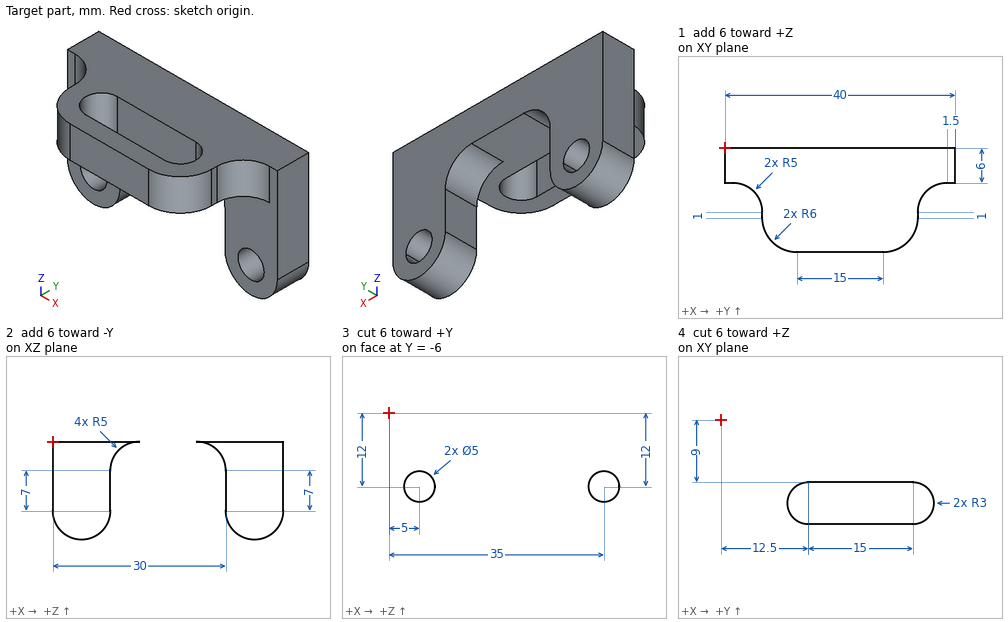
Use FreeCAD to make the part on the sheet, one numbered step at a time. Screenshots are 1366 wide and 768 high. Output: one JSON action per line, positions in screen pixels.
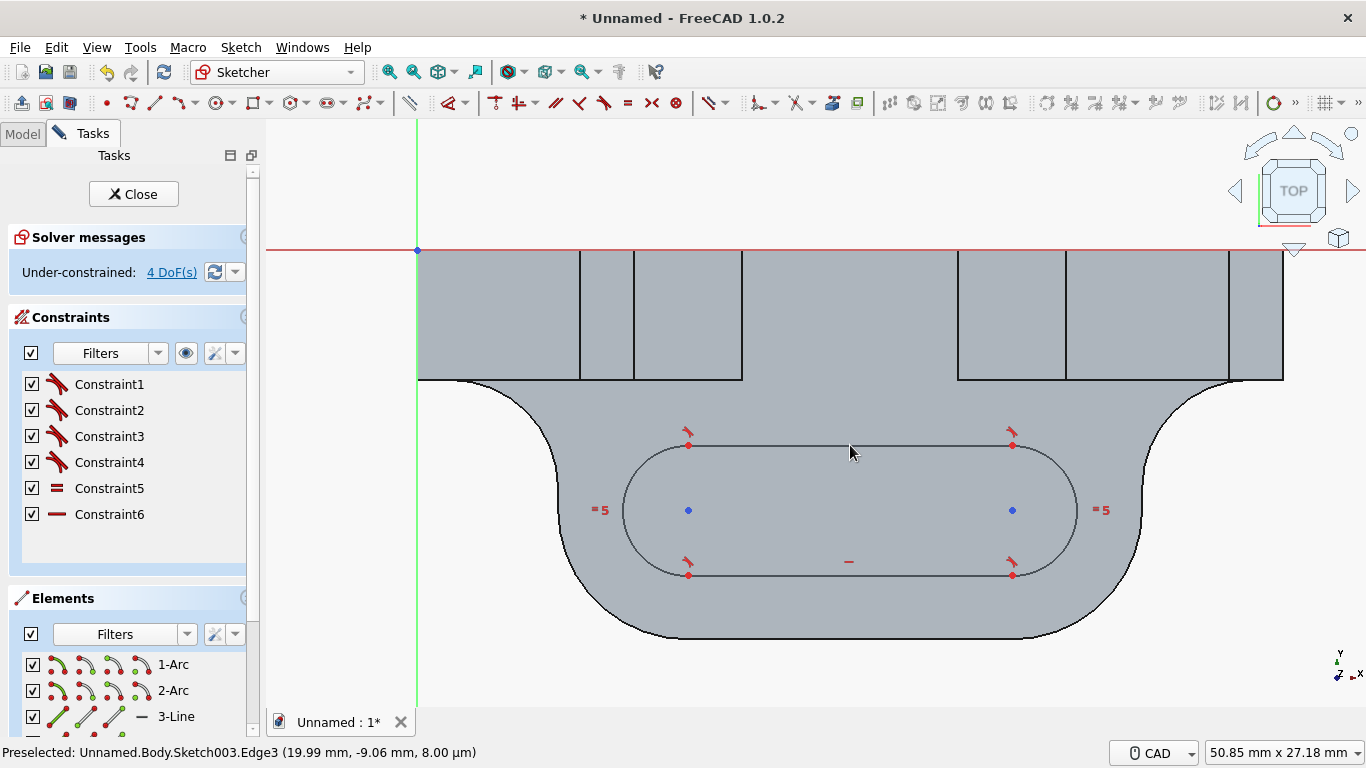
{"action": "key", "text": "d"}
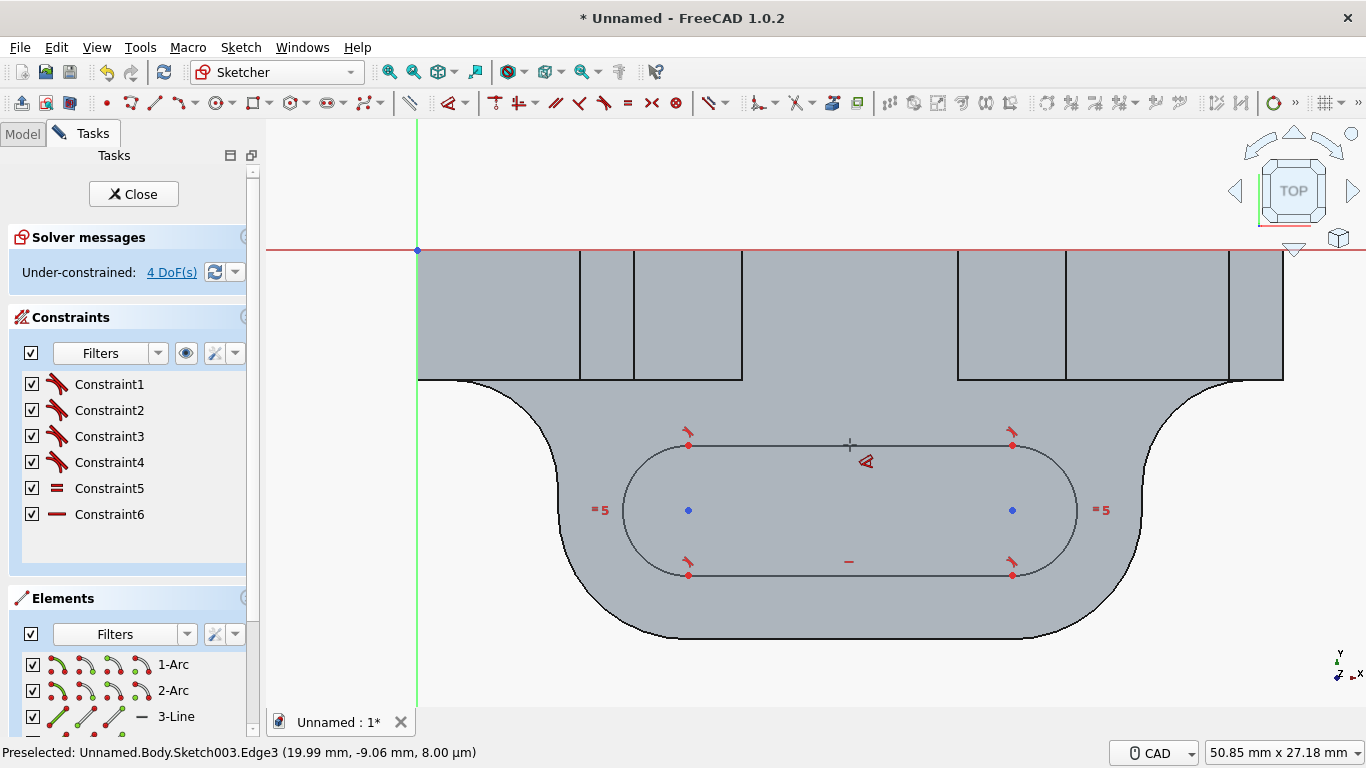
{"action": "left_click", "coordinate": [635, 473]}
{"action": "left_click", "coordinate": [609, 454]}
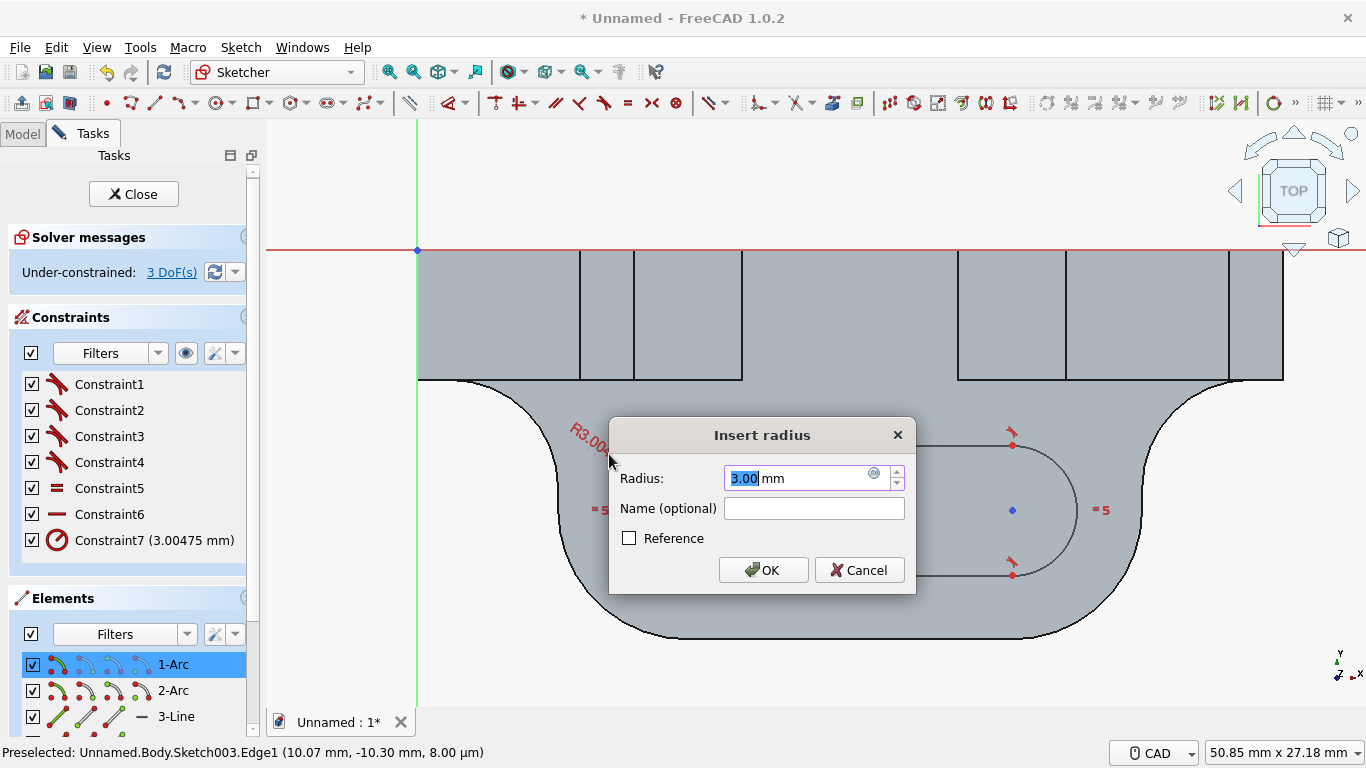
{"action": "type", "text": "3"}
{"action": "key", "text": "Return"}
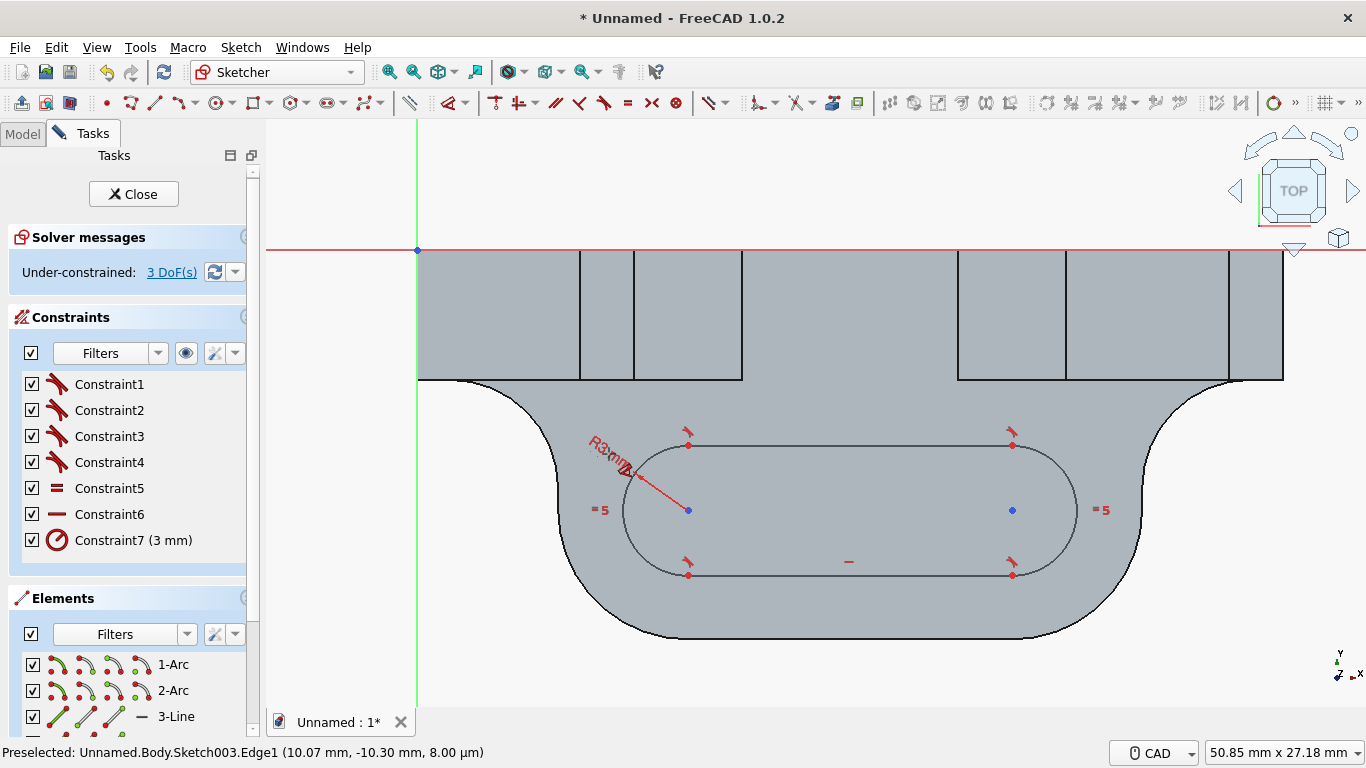
{"action": "left_click", "coordinate": [785, 446]}
{"action": "left_click", "coordinate": [850, 480]}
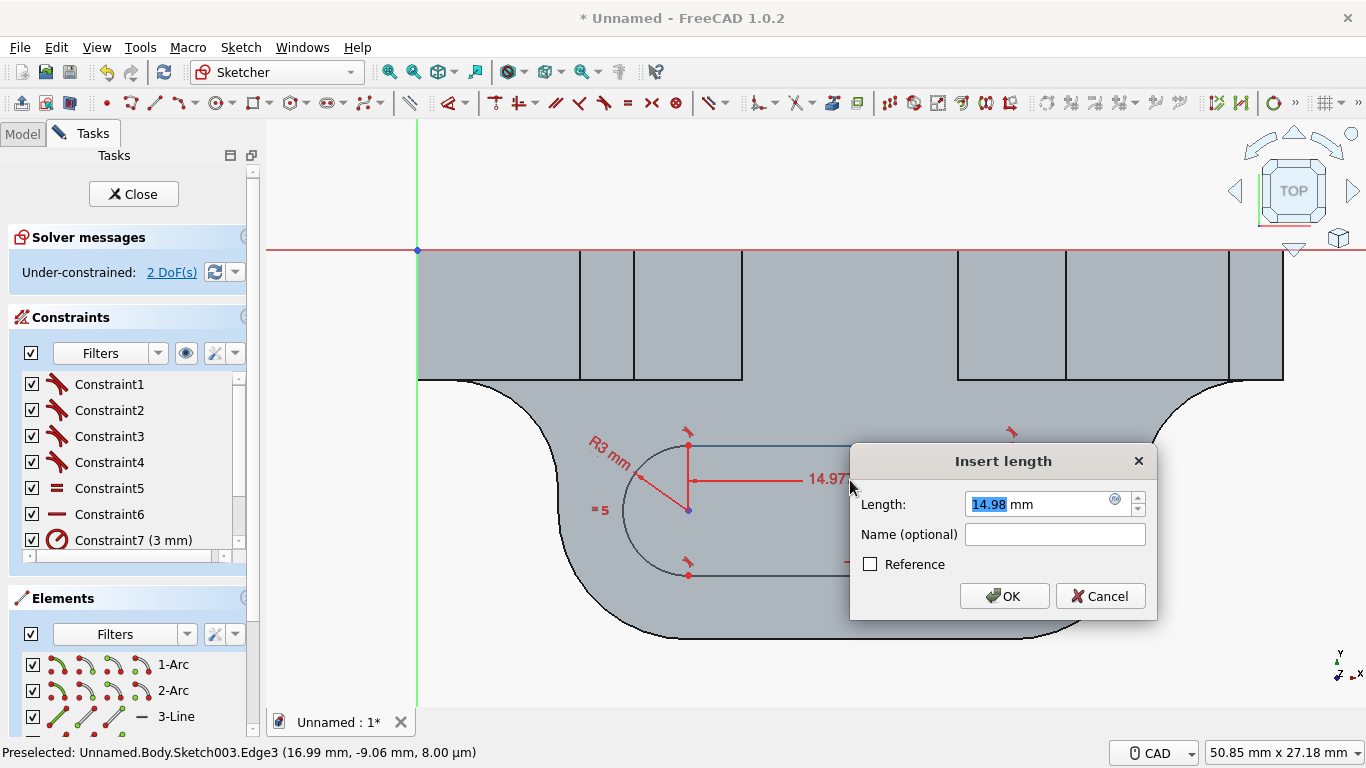
{"action": "type", "text": "15"}
{"action": "key", "text": "Return"}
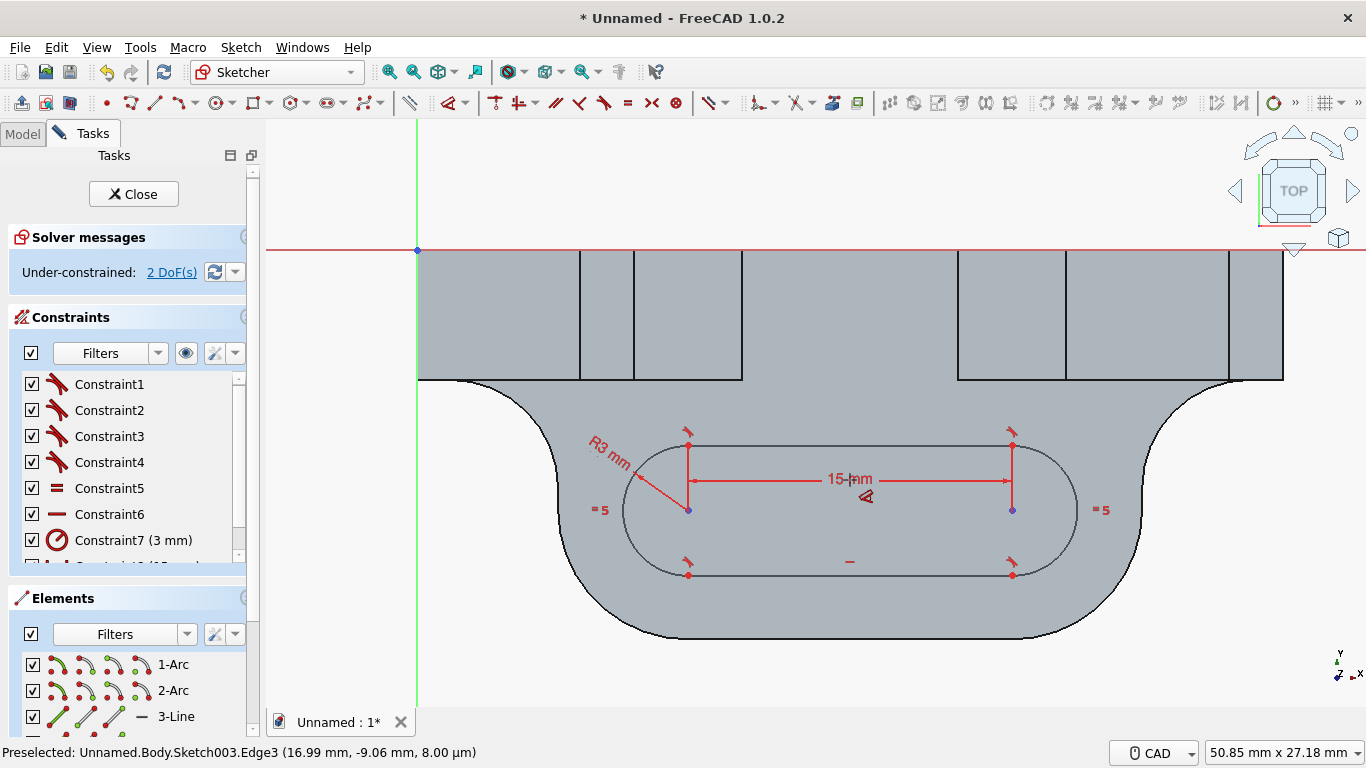
{"action": "left_click", "coordinate": [688, 446]}
{"action": "left_click", "coordinate": [384, 348]}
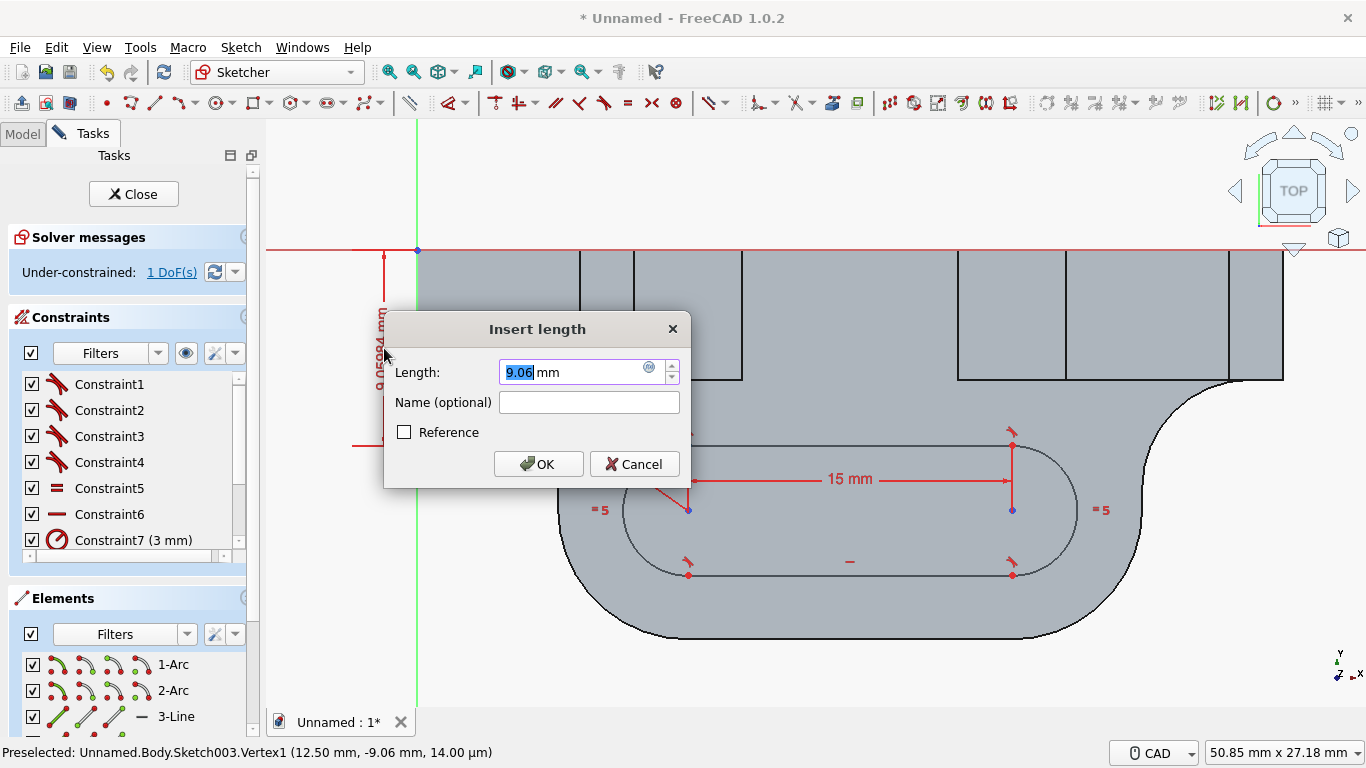
{"action": "type", "text": "9"}
{"action": "key", "text": "Return"}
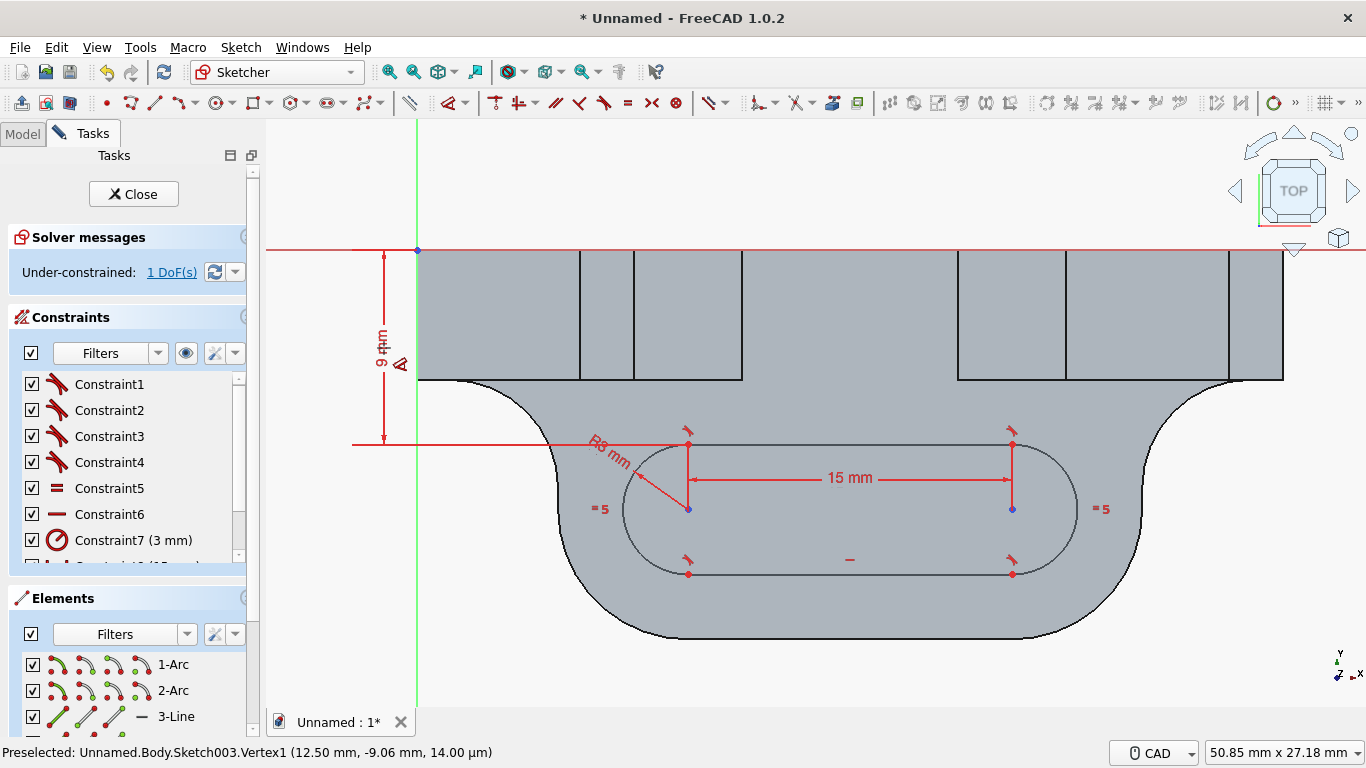
{"action": "left_click", "coordinate": [688, 445]}
{"action": "left_click", "coordinate": [553, 216]}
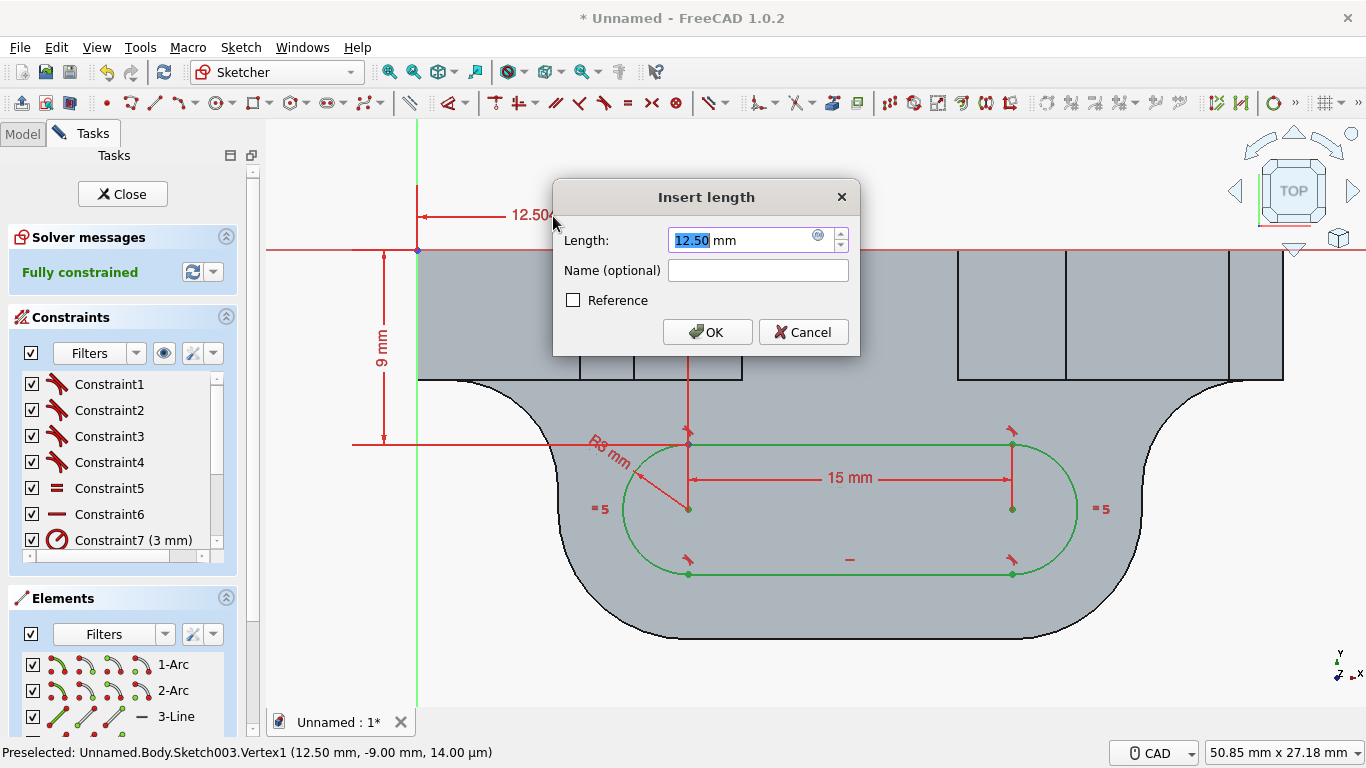
{"action": "type", "text": "12.5"}
{"action": "key", "text": "Return"}
{"action": "key", "text": "Escape"}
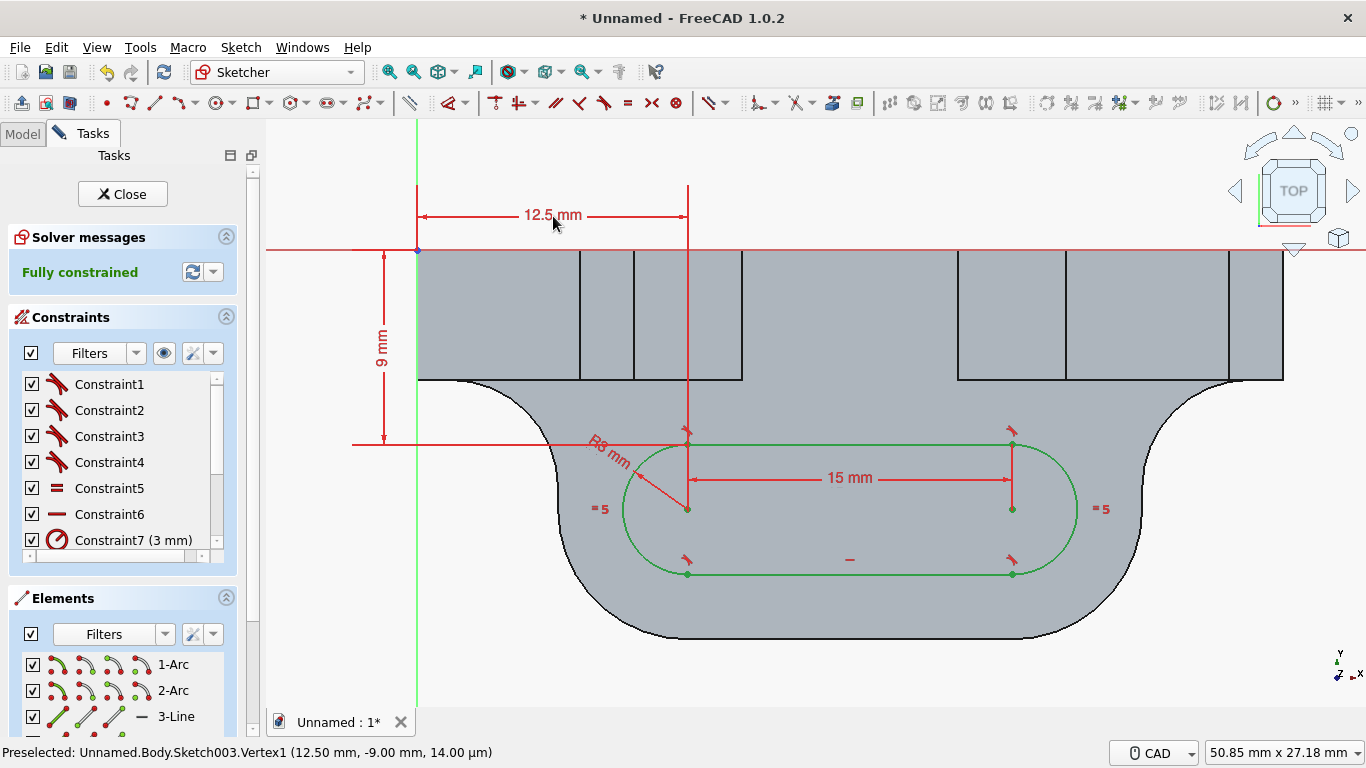
{"action": "left_click", "coordinate": [123, 194]}